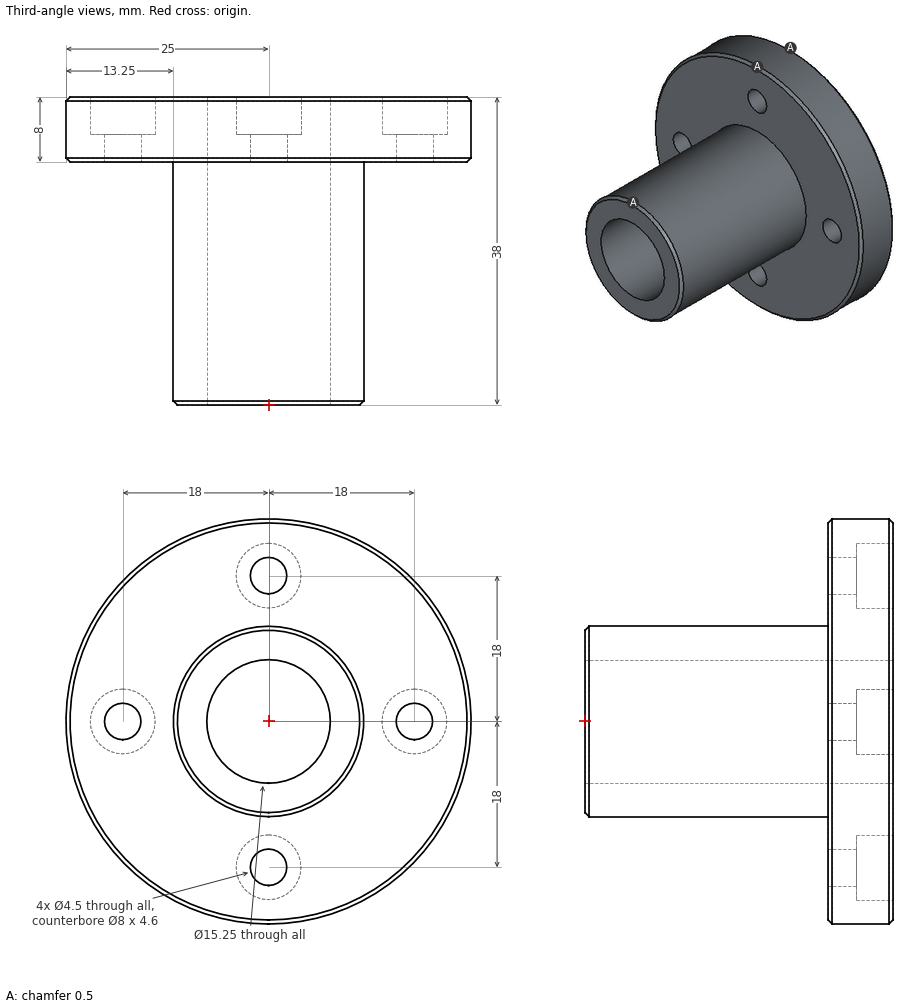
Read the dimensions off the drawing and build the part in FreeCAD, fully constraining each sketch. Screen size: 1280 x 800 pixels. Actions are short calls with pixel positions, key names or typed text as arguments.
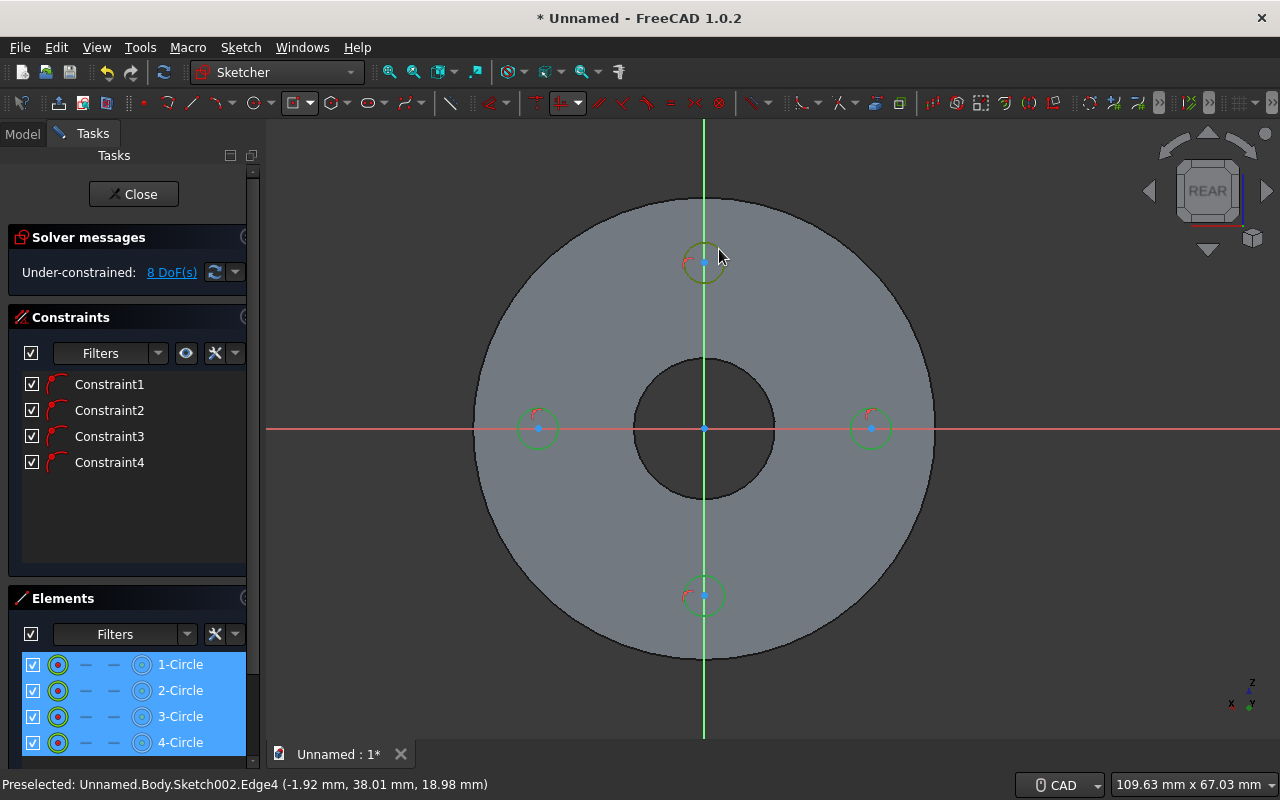
click(672, 104)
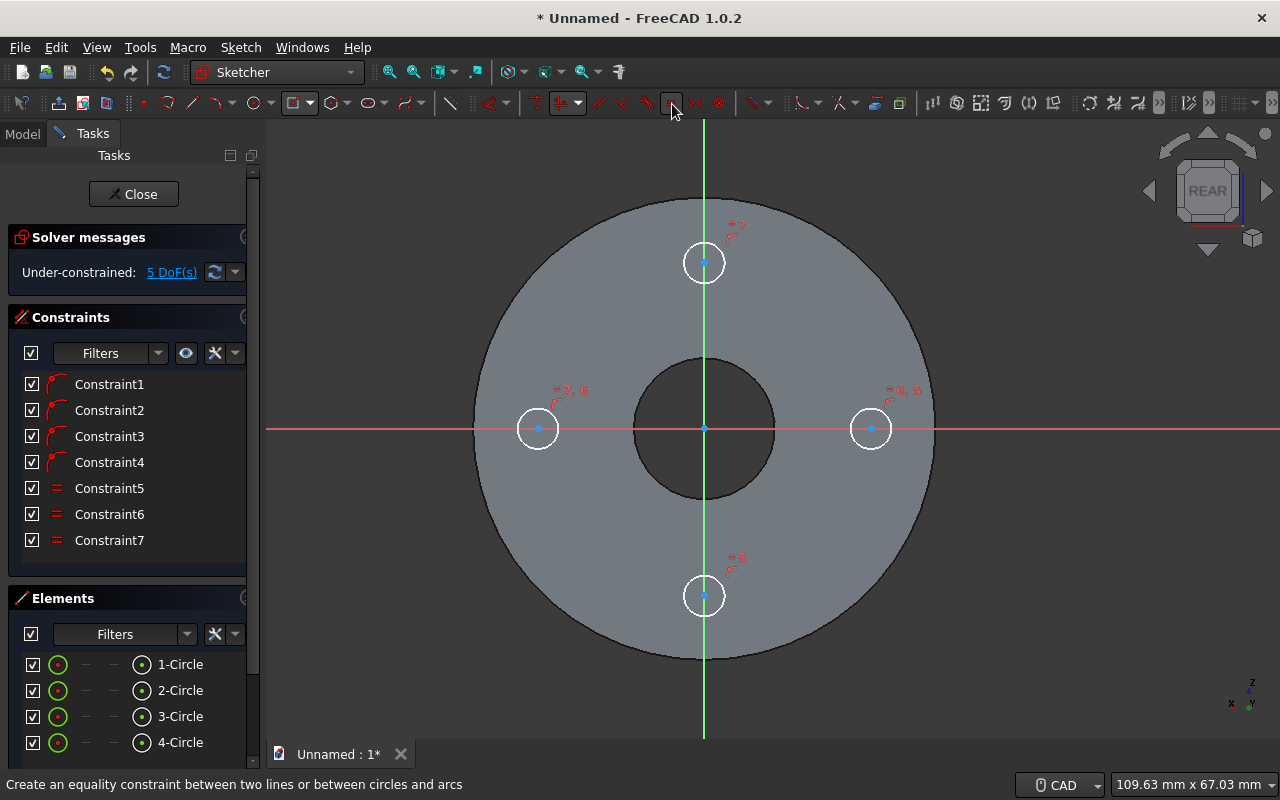
key(d)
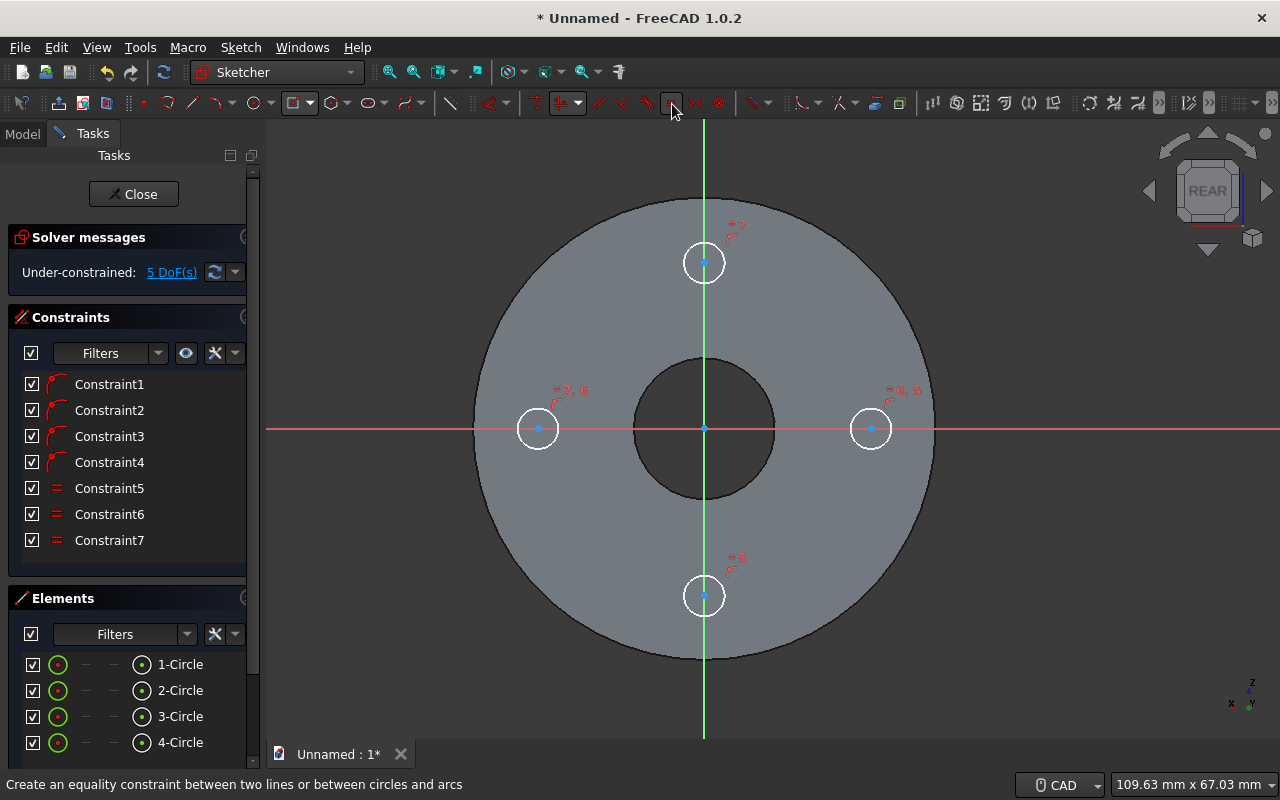
click(719, 582)
click(742, 560)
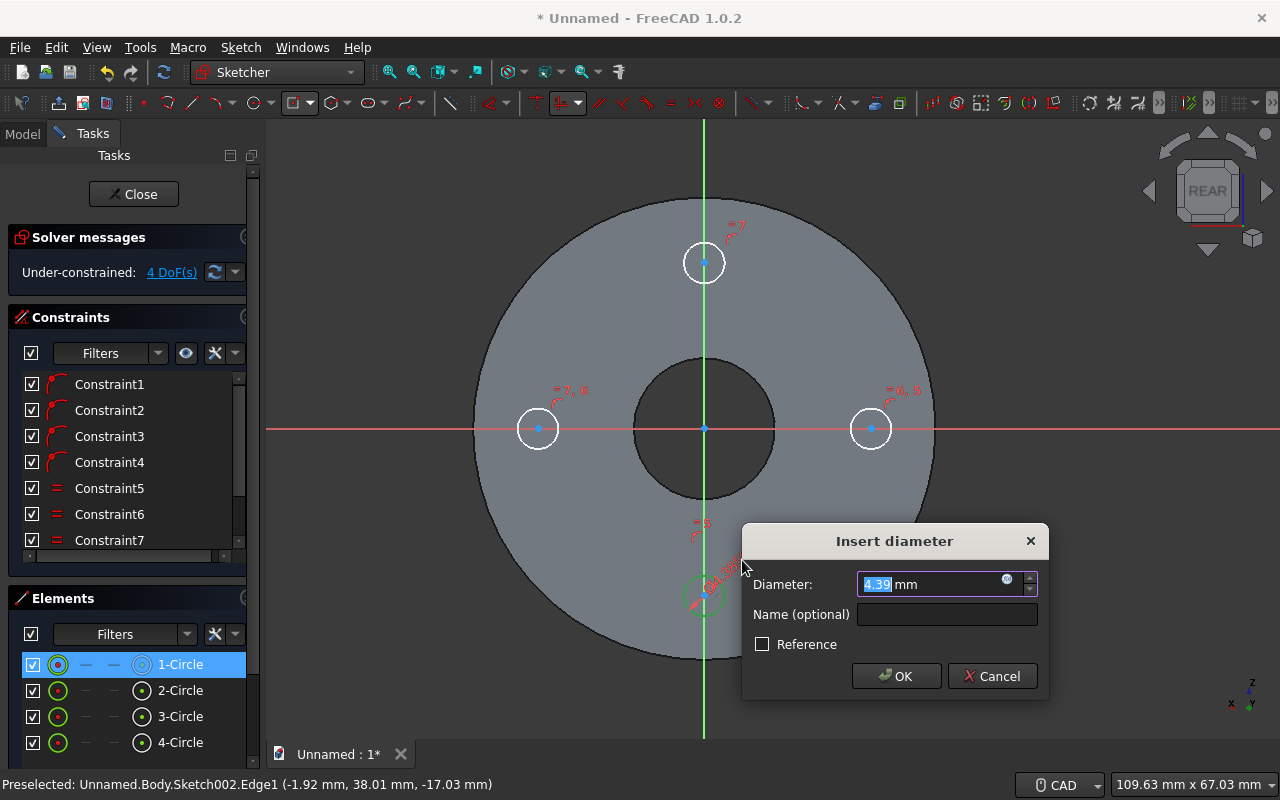
text(4.5)
key(Return)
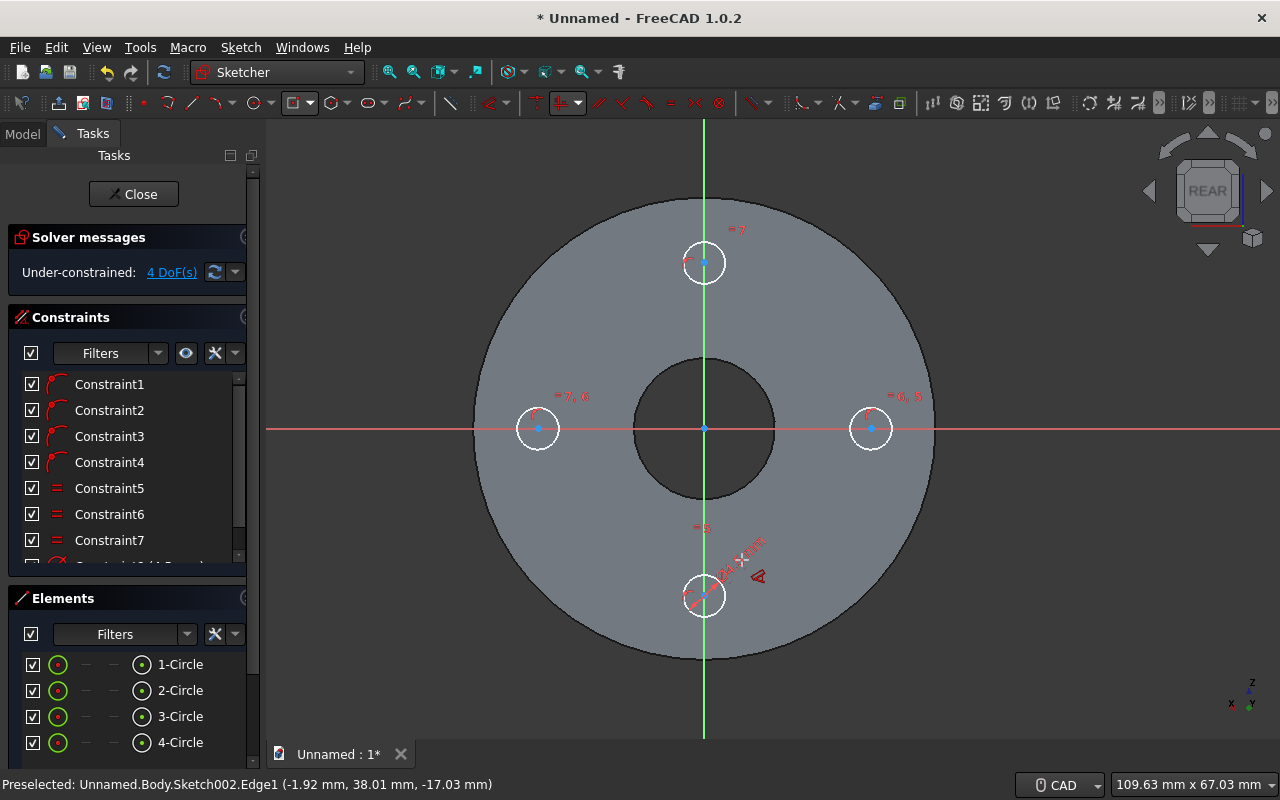
click(704, 596)
click(738, 512)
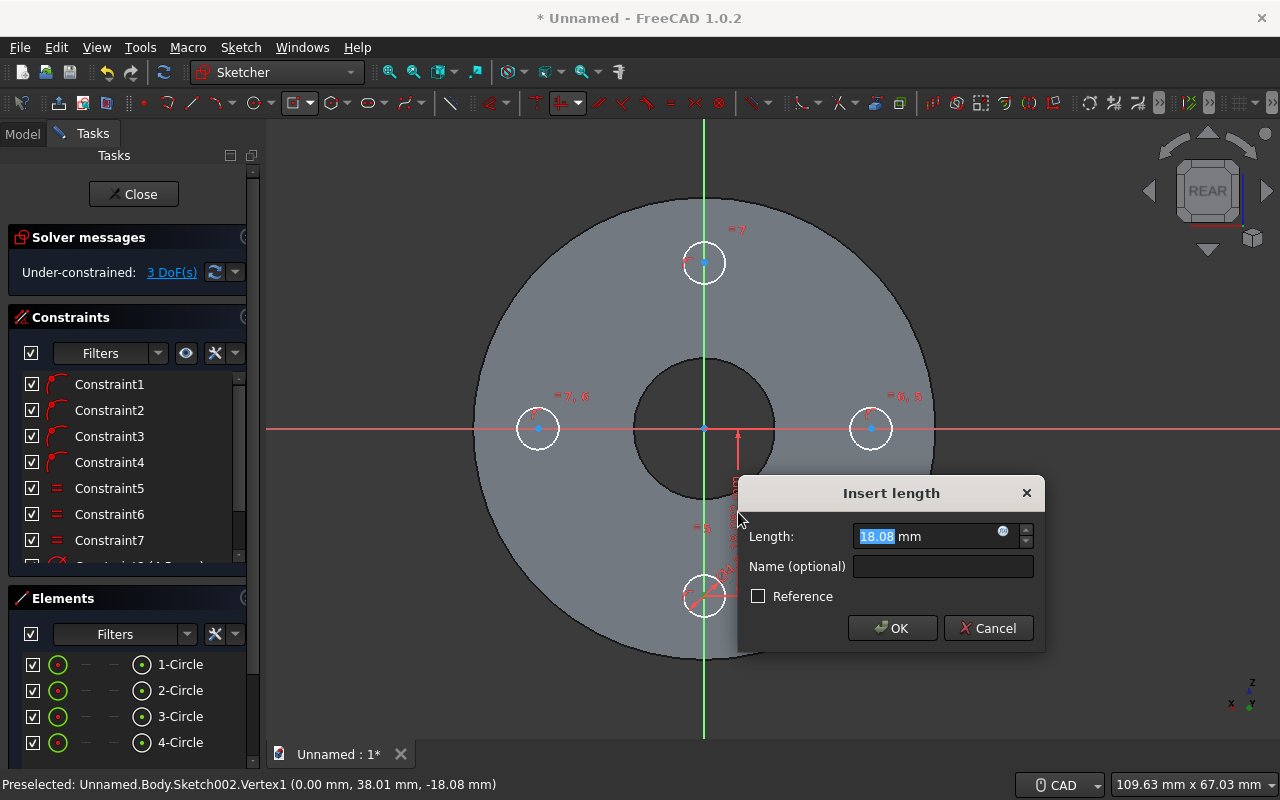
text(18)
key(Return)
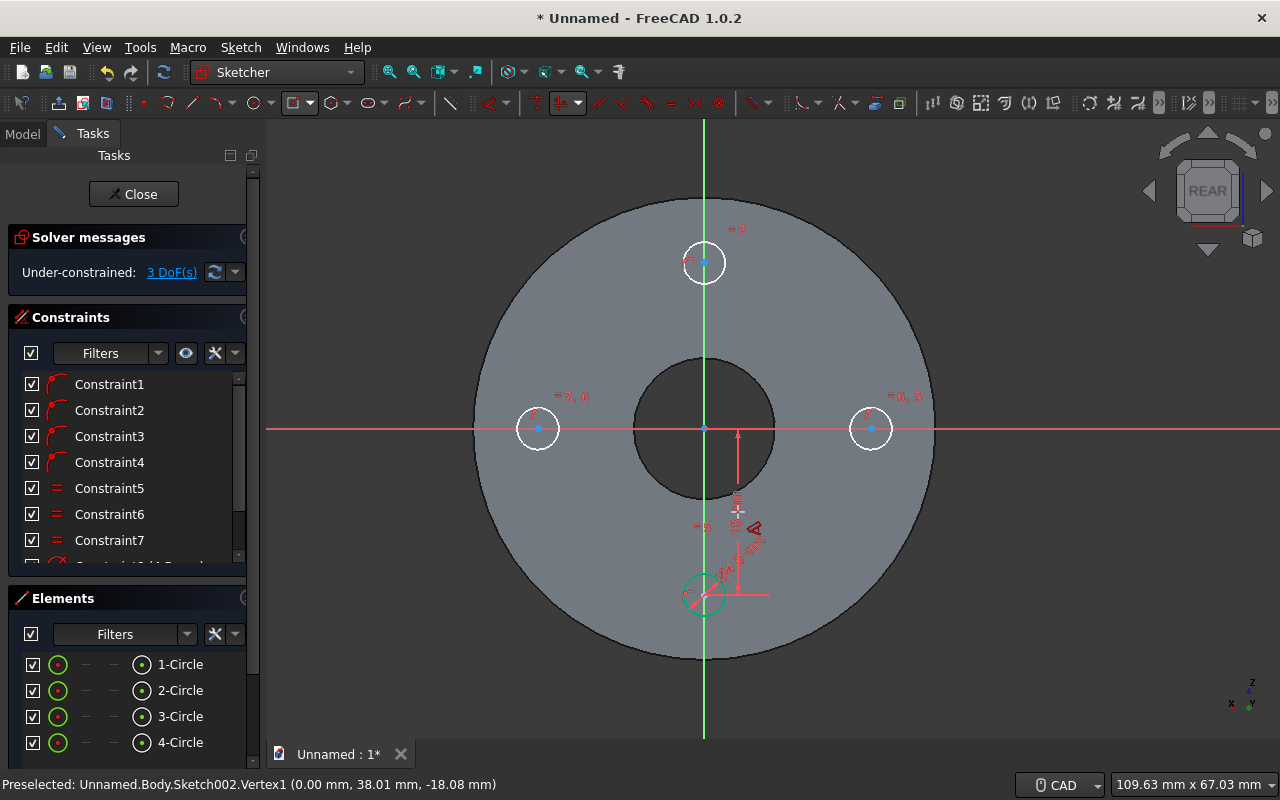
click(871, 429)
click(788, 463)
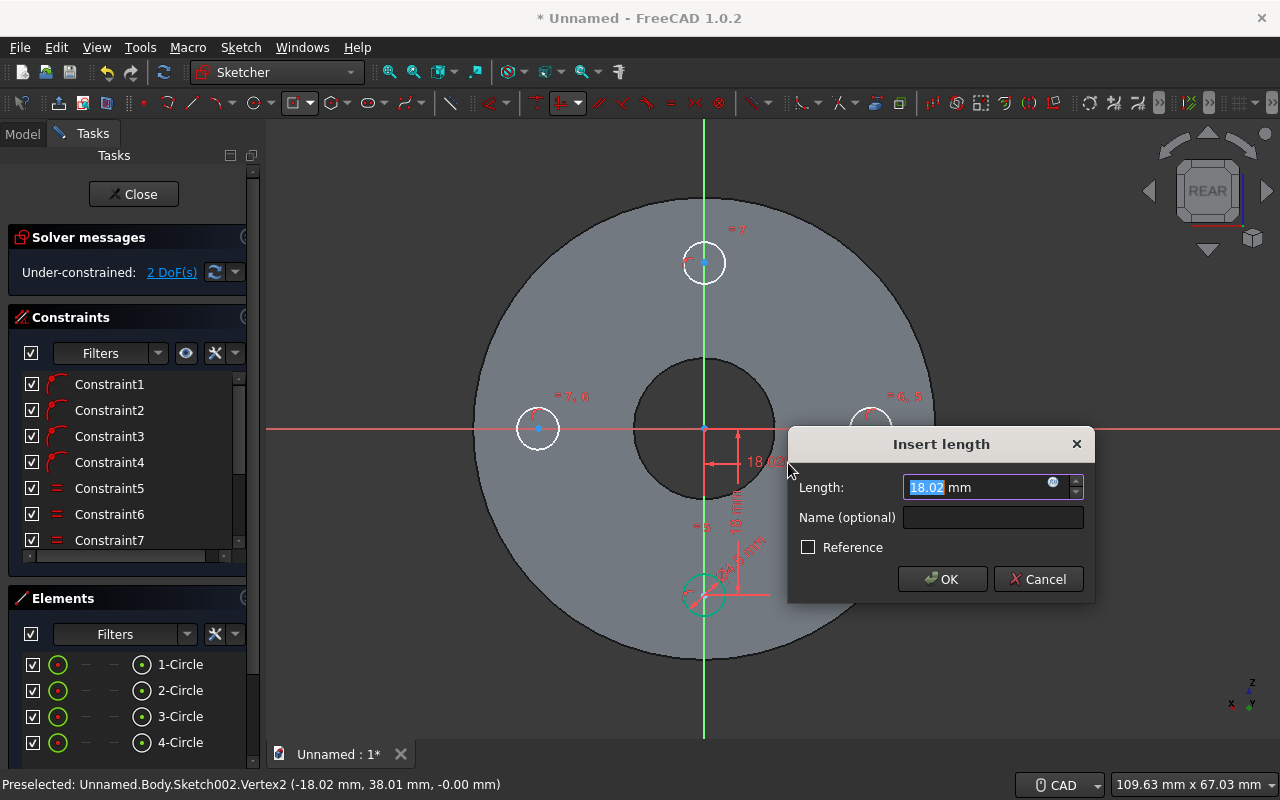
text(18)
key(Return)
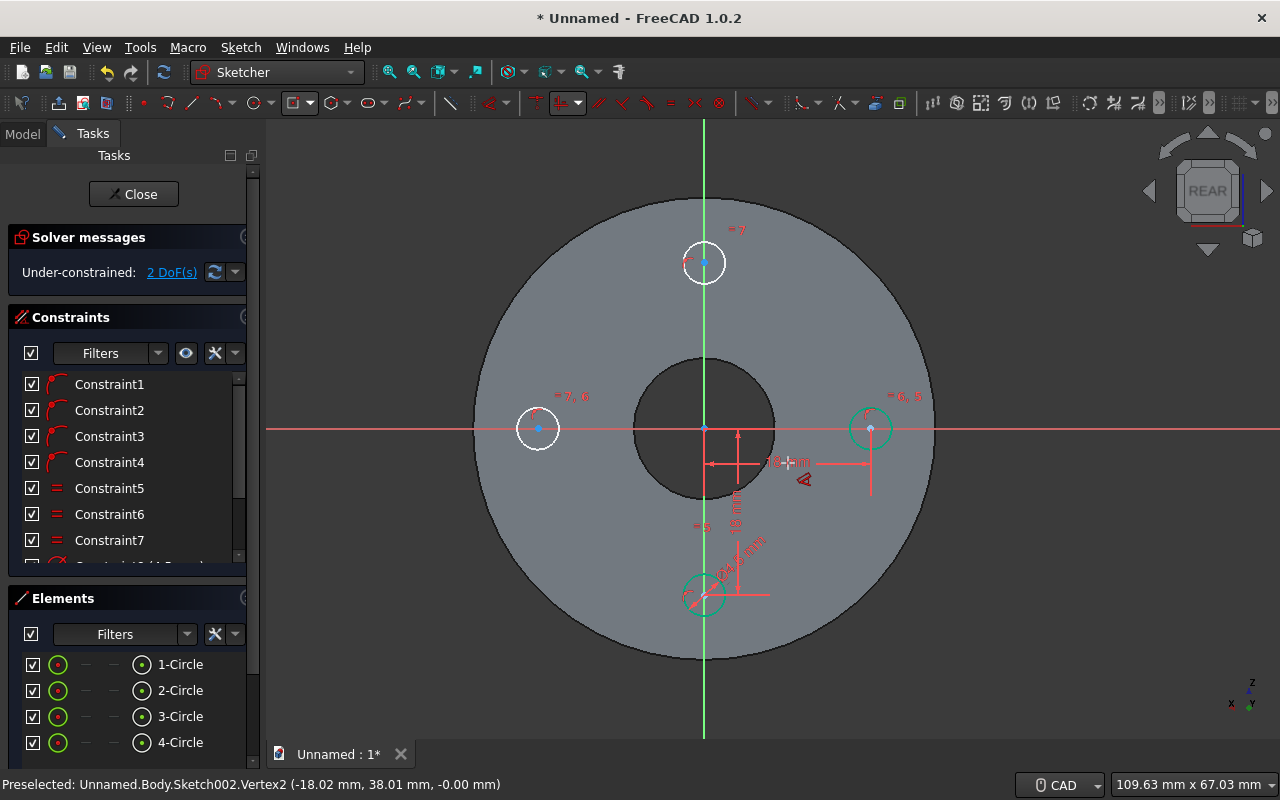
click(538, 429)
click(621, 463)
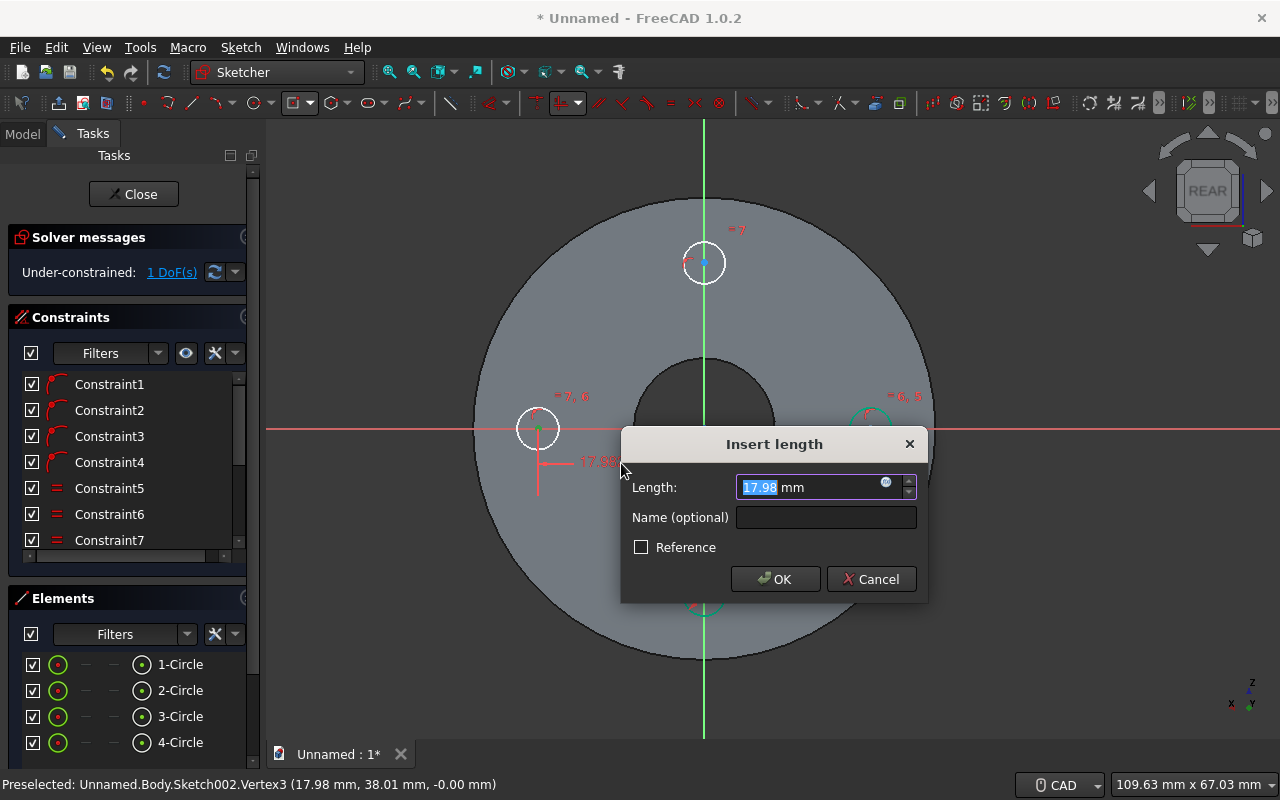
text(18)
key(Return)